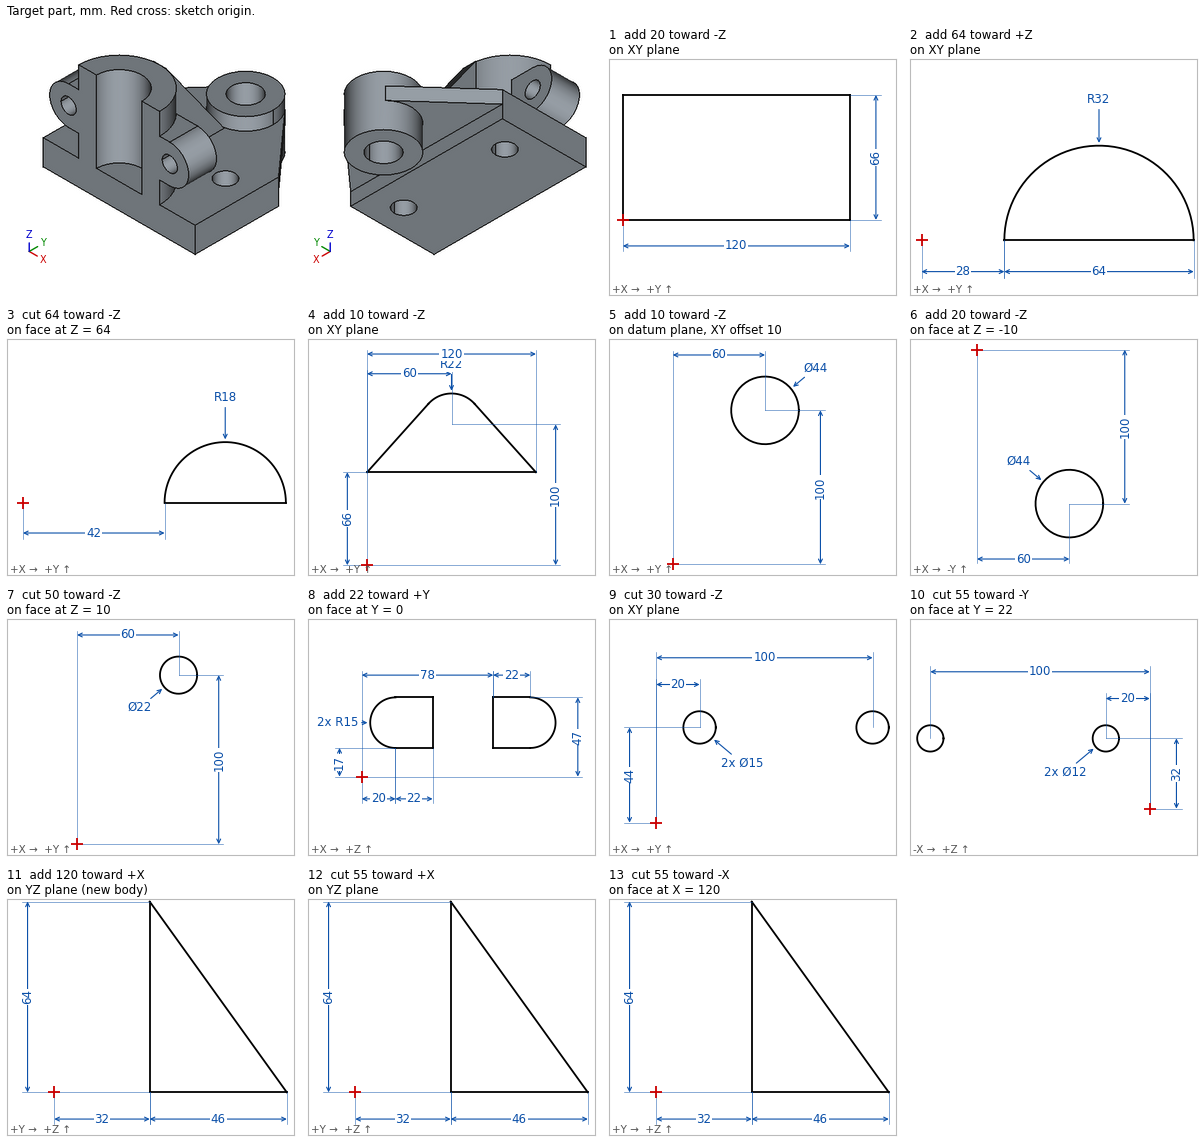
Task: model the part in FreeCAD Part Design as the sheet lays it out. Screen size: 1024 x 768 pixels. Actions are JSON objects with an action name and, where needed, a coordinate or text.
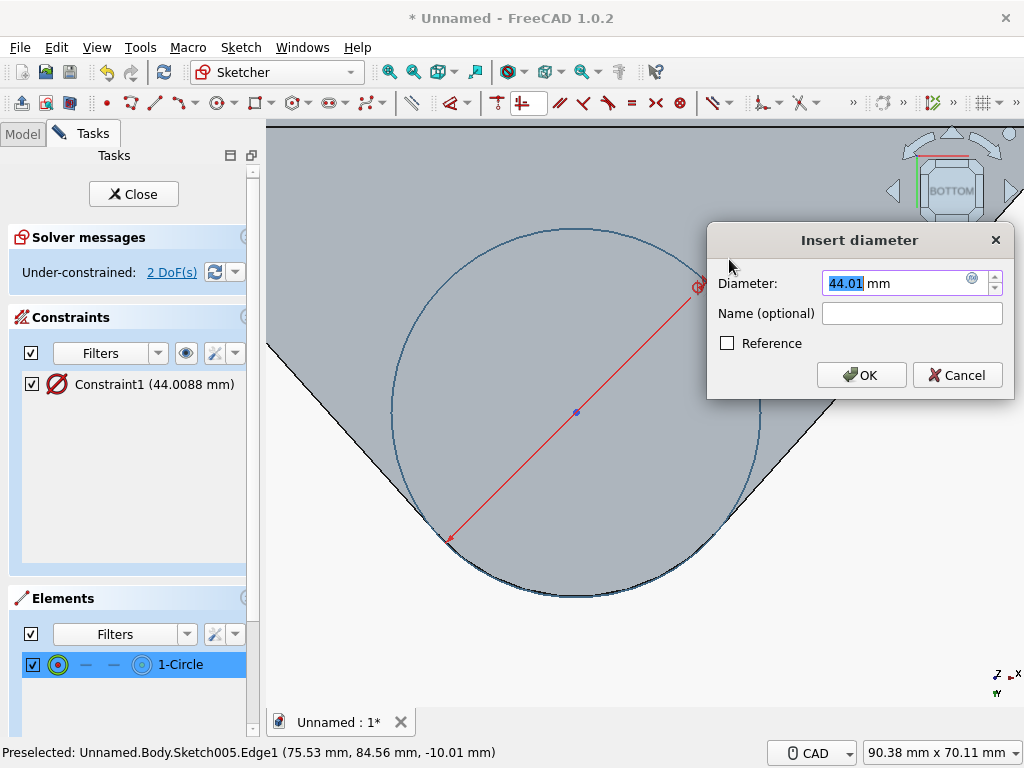
{"action": "type", "text": "44"}
{"action": "key", "text": "Return"}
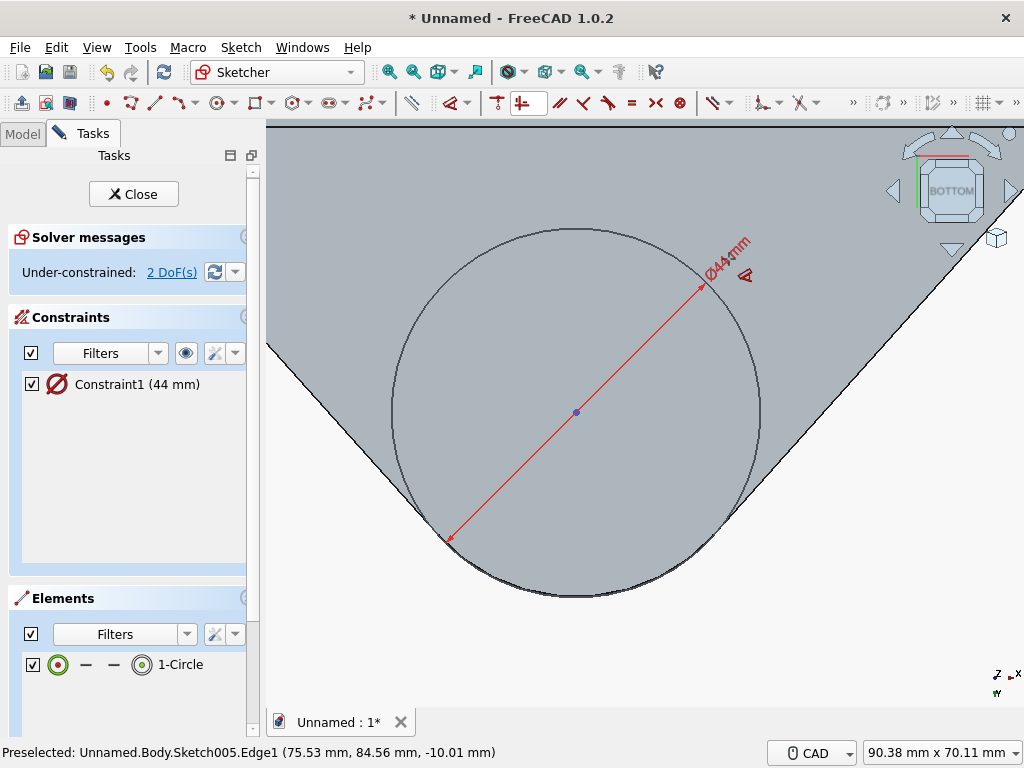
{"action": "left_click", "coordinate": [576, 413]}
{"action": "left_click", "coordinate": [435, 447]}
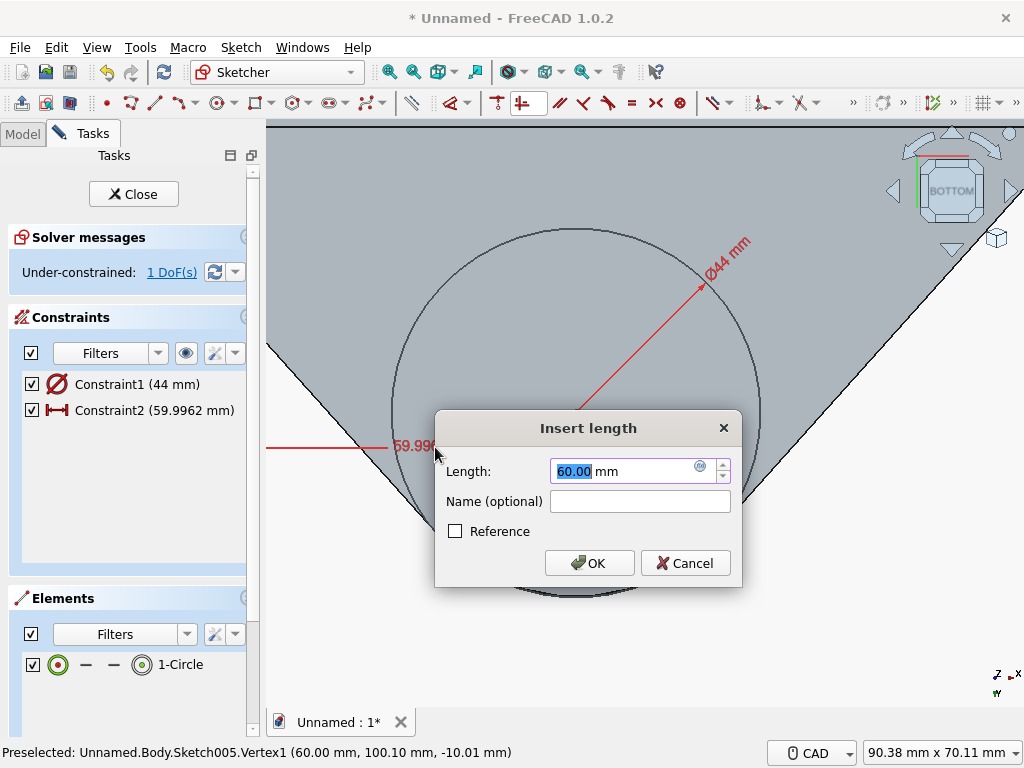
{"action": "type", "text": "60"}
{"action": "key", "text": "Return"}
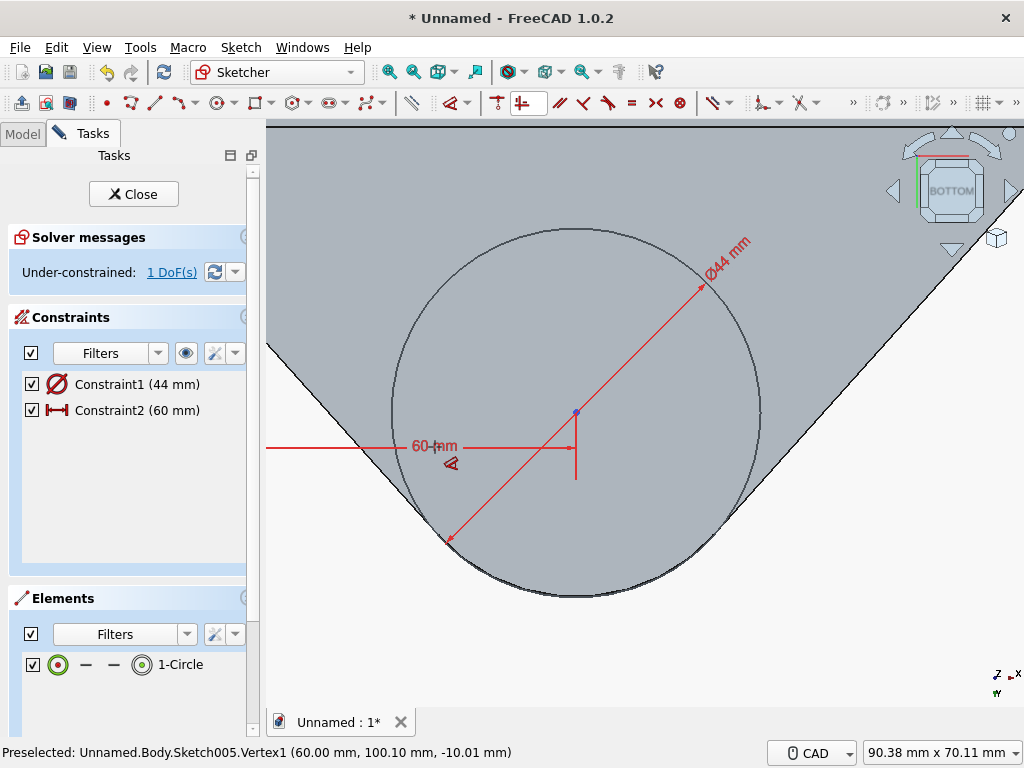
{"action": "left_click", "coordinate": [576, 413]}
{"action": "left_click", "coordinate": [610, 280]}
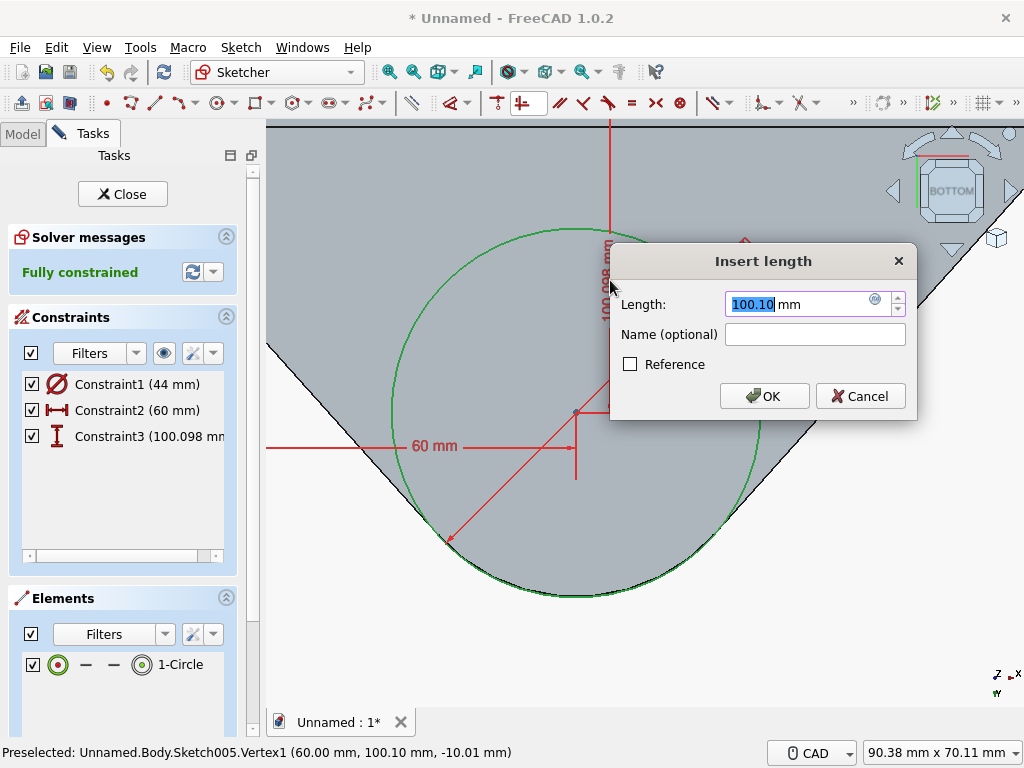
{"action": "type", "text": "100"}
{"action": "key", "text": "Return"}
{"action": "key", "text": "Escape"}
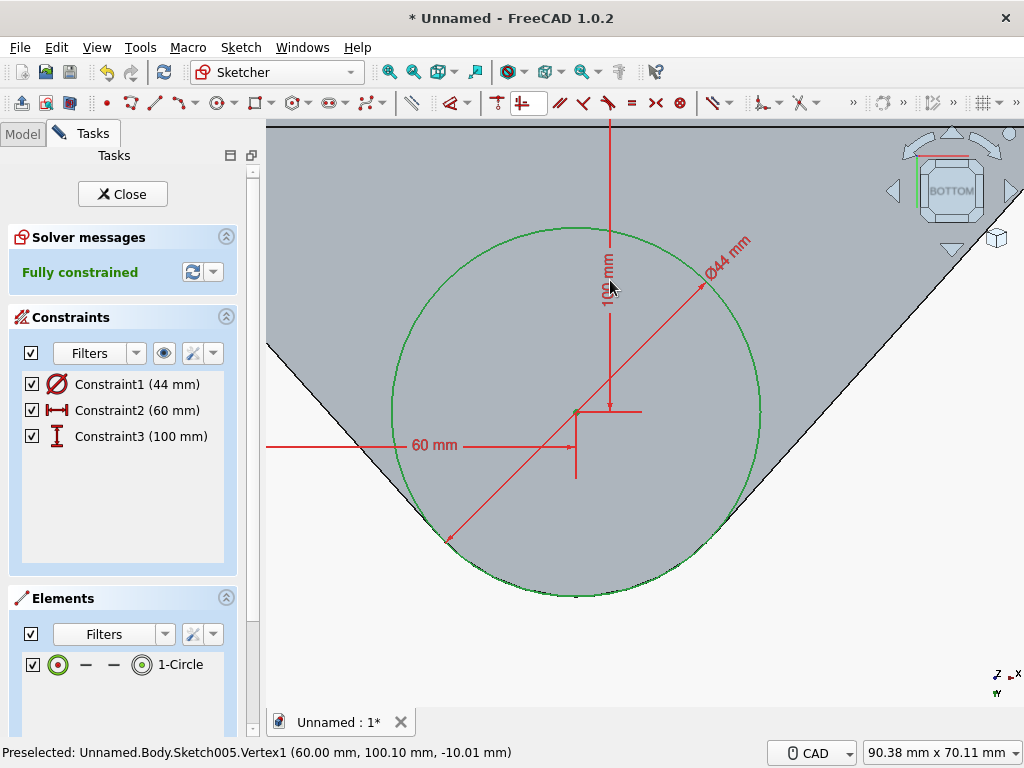
{"action": "left_click", "coordinate": [123, 194]}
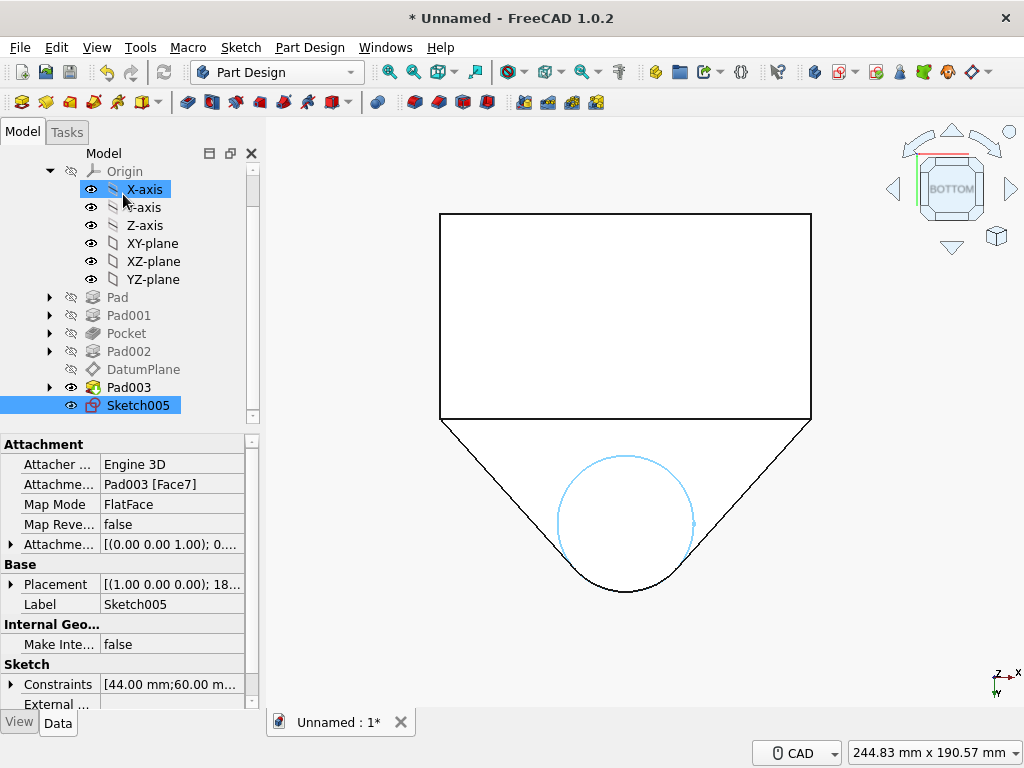
{"action": "left_click", "coordinate": [22, 102]}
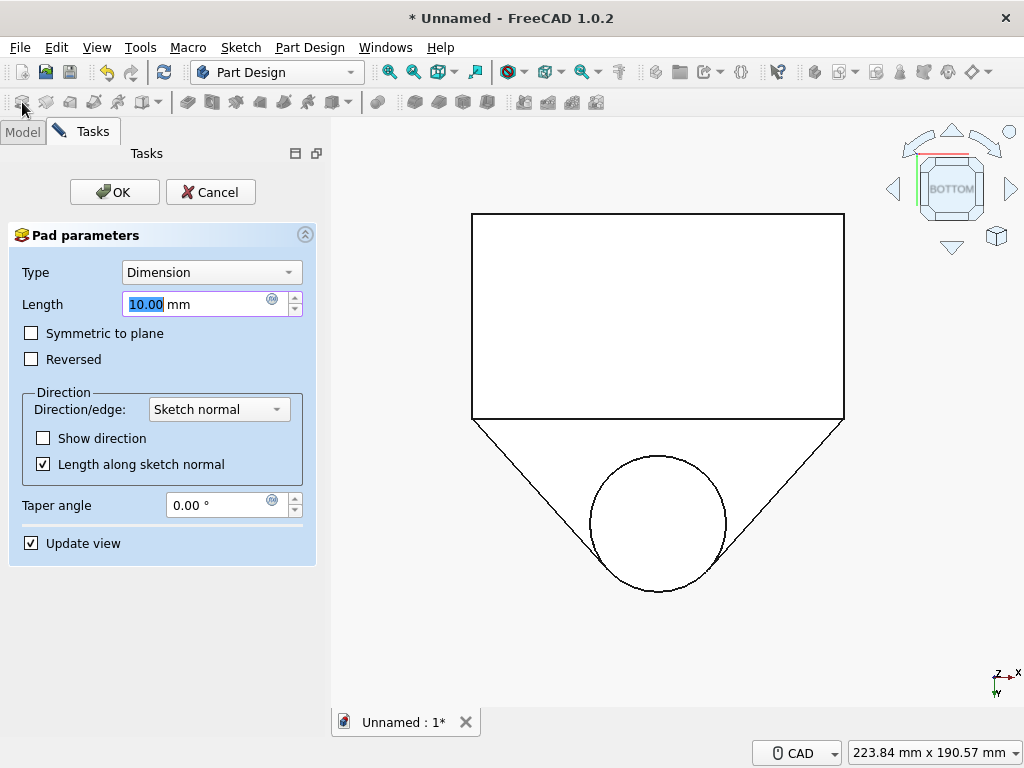
{"action": "type", "text": "20"}
{"action": "key", "text": "Tab"}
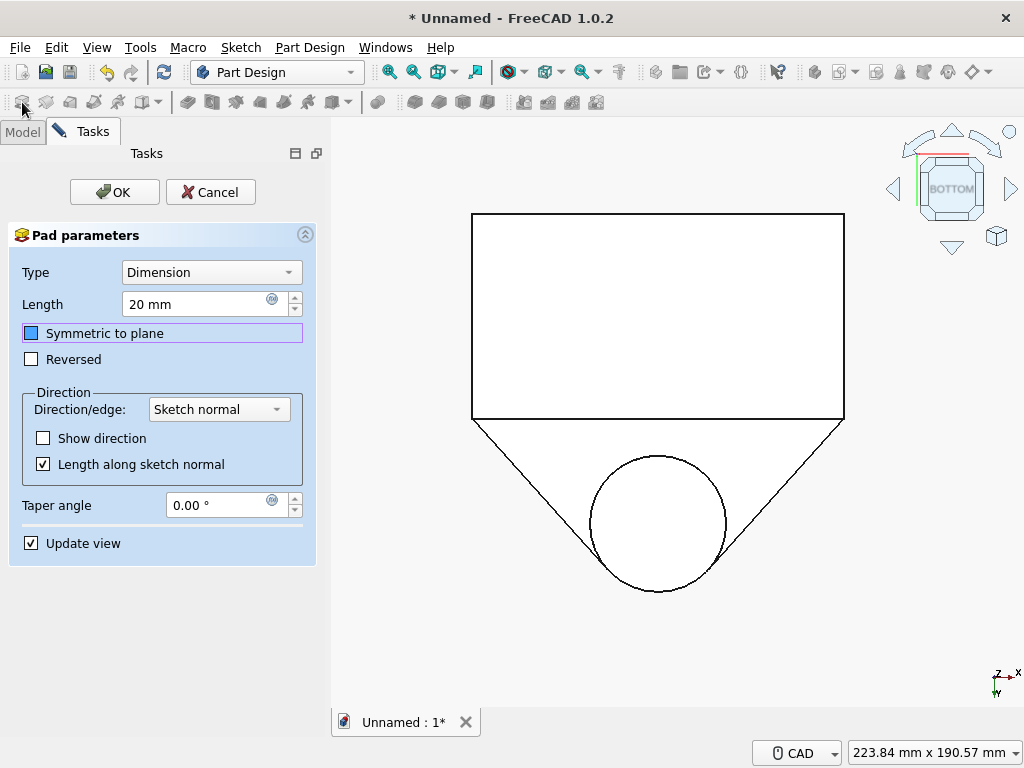
{"action": "left_click", "coordinate": [115, 192]}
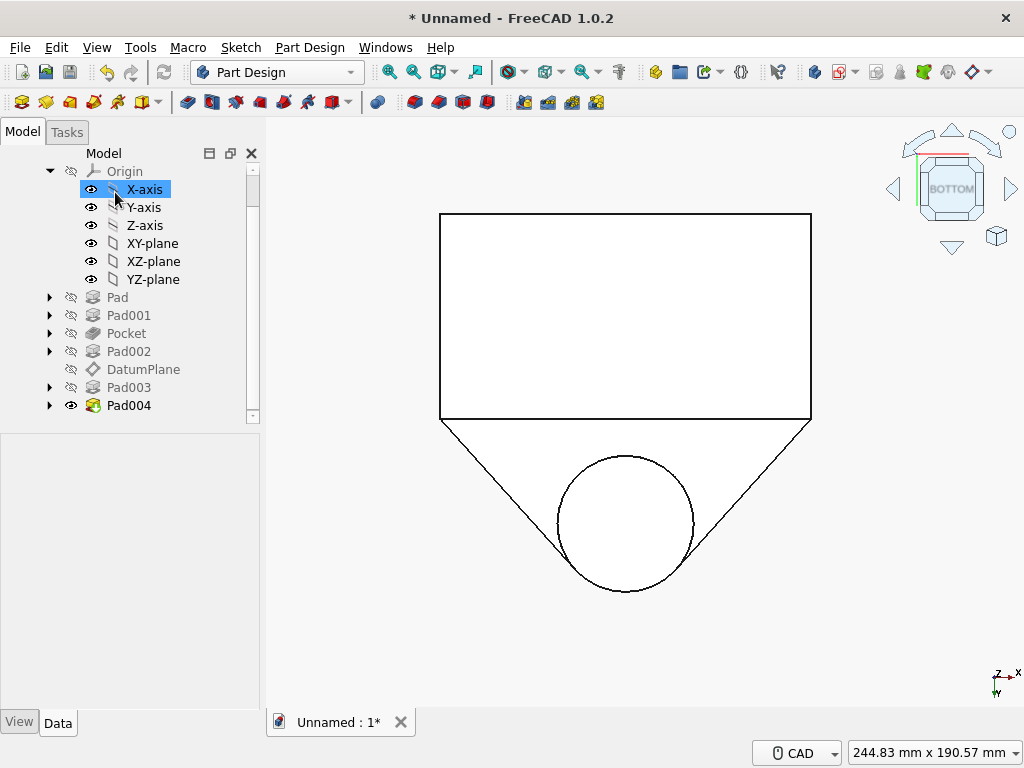
{"action": "key", "text": "0"}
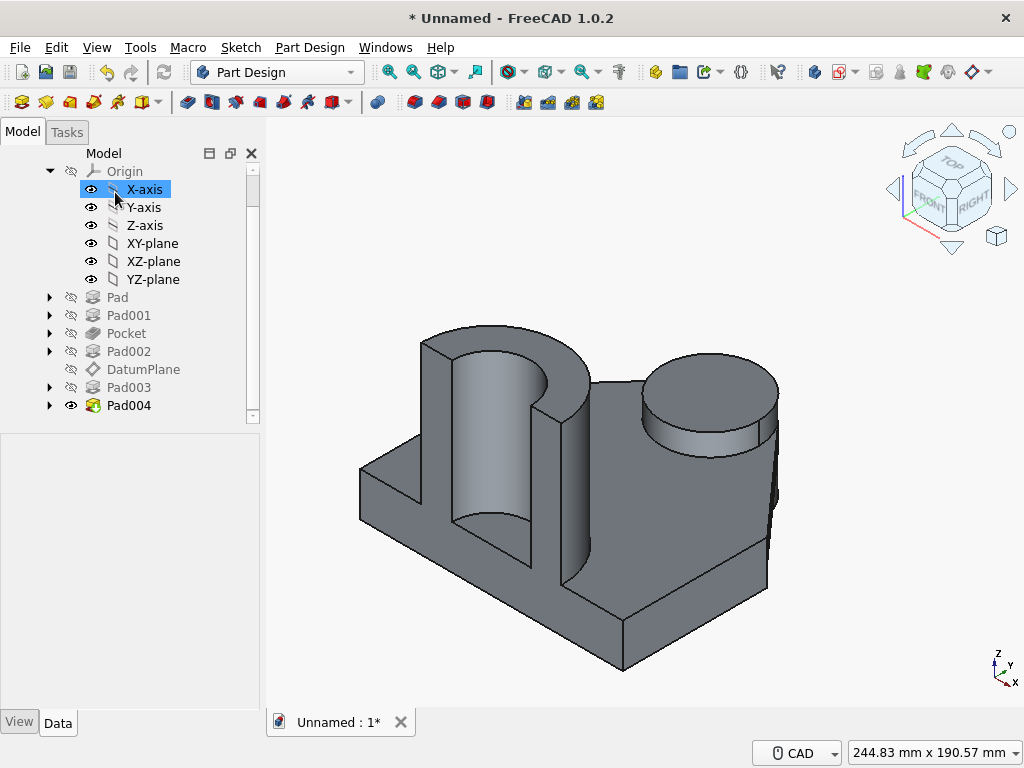
{"action": "left_click", "coordinate": [710, 392]}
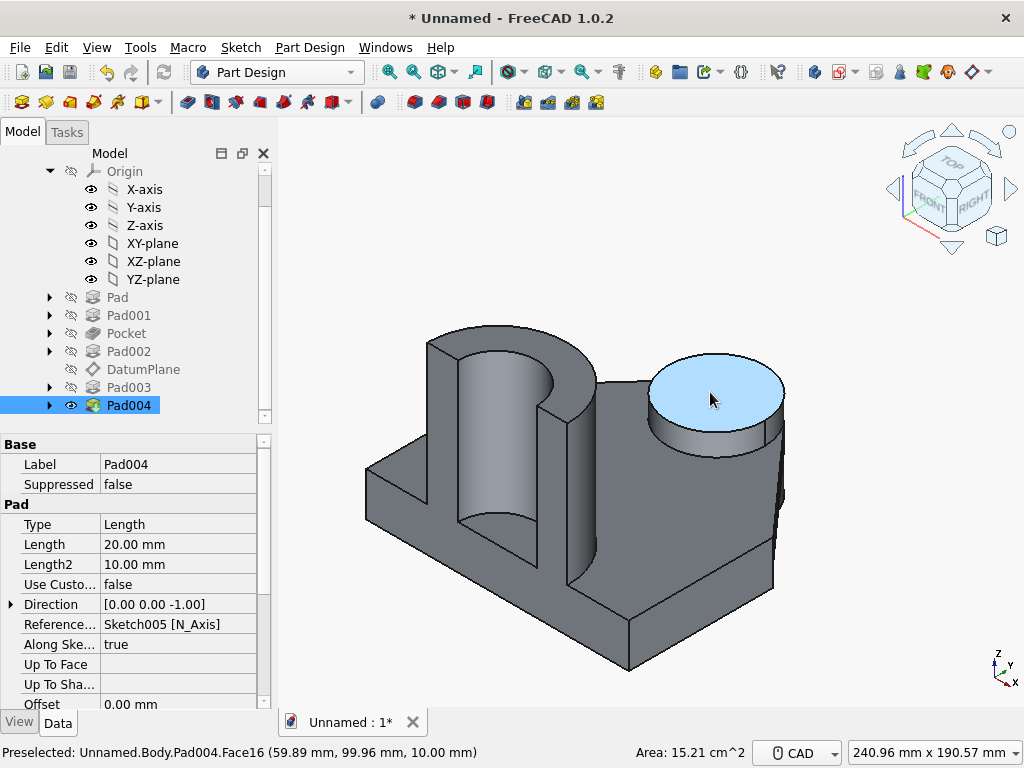
{"action": "left_click", "coordinate": [840, 72]}